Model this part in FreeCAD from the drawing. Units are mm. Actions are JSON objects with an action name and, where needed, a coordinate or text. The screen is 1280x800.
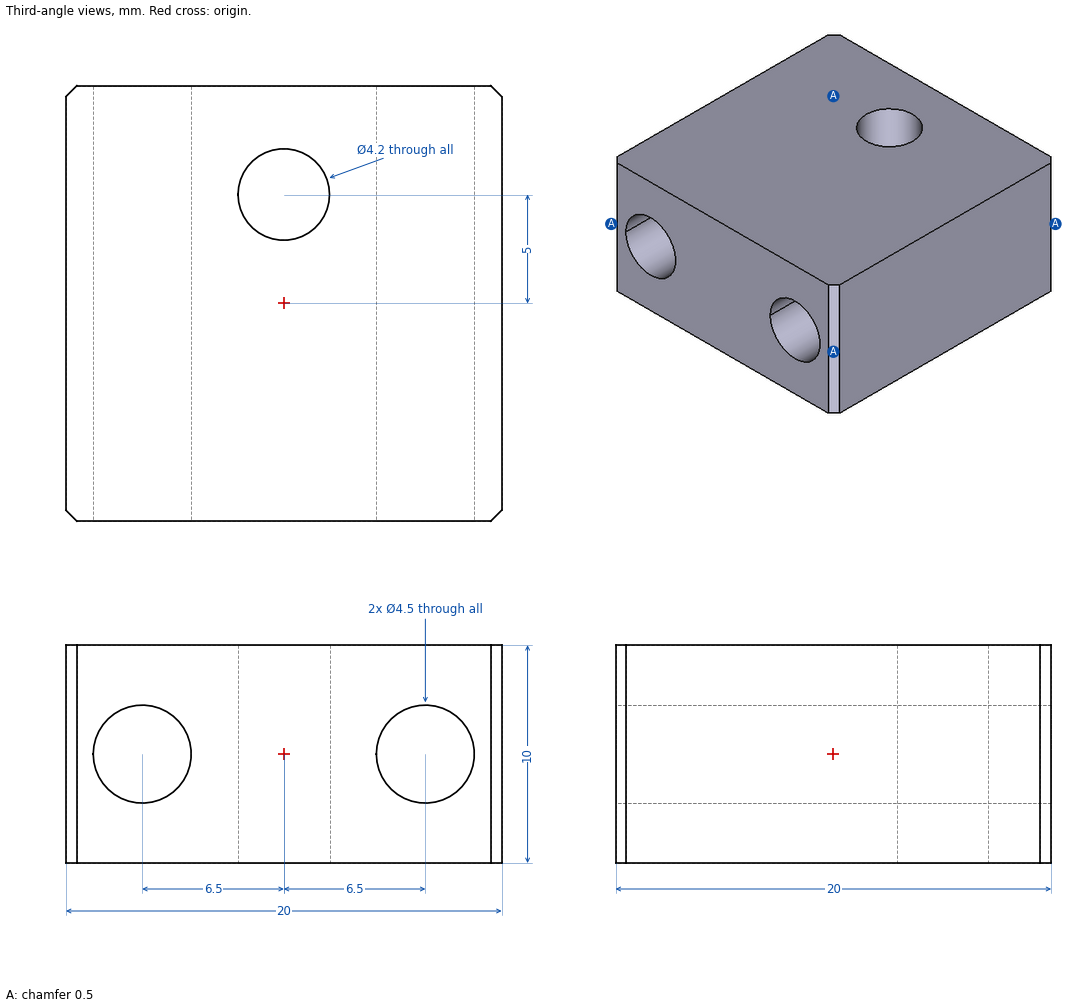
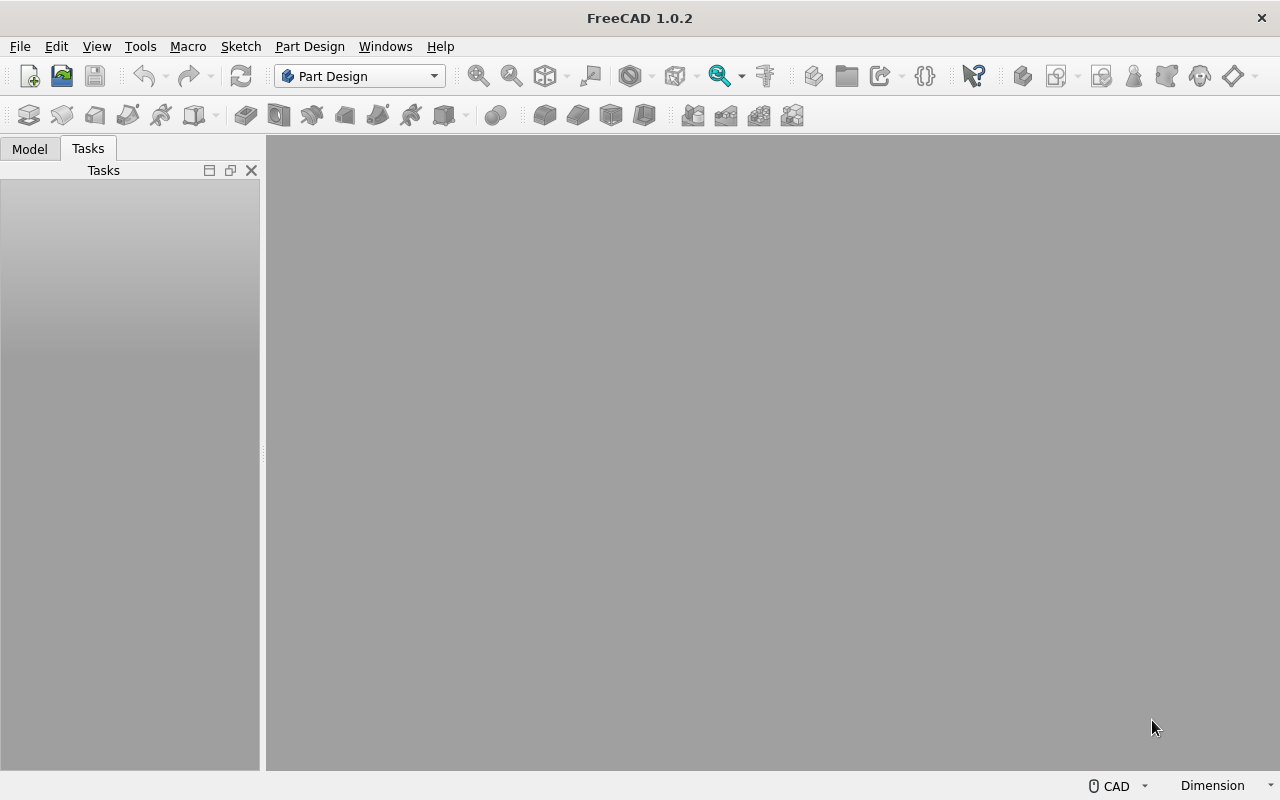
{"action": "key", "text": "ctrl+n"}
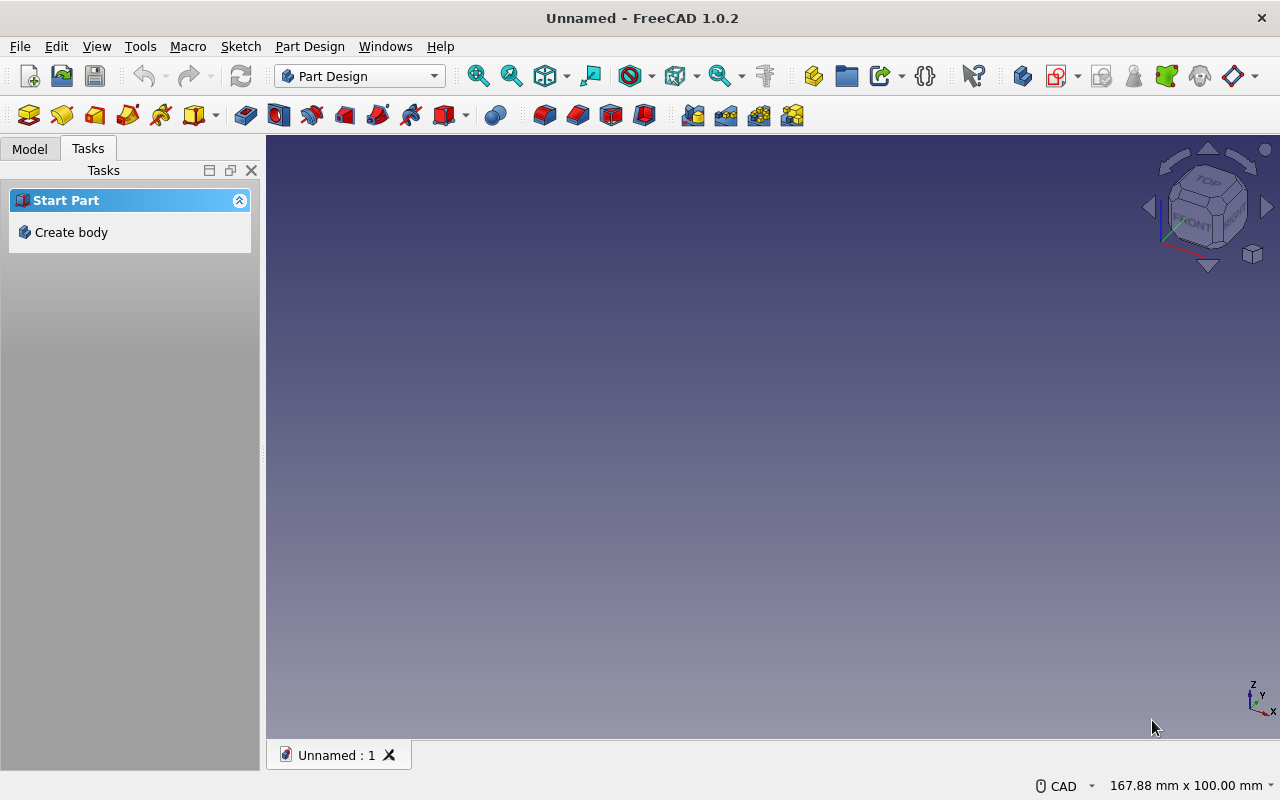
{"action": "left_click", "coordinate": [1056, 76]}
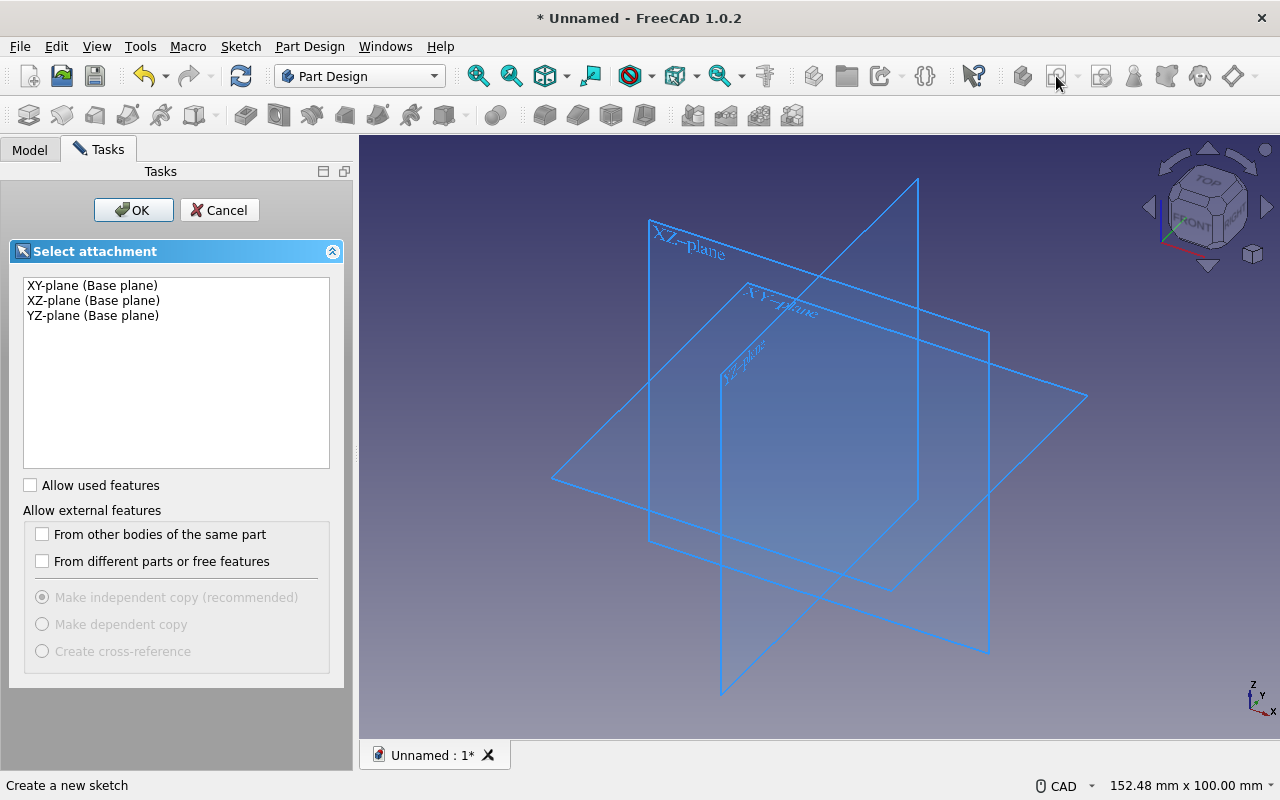
{"action": "left_click", "coordinate": [84, 300]}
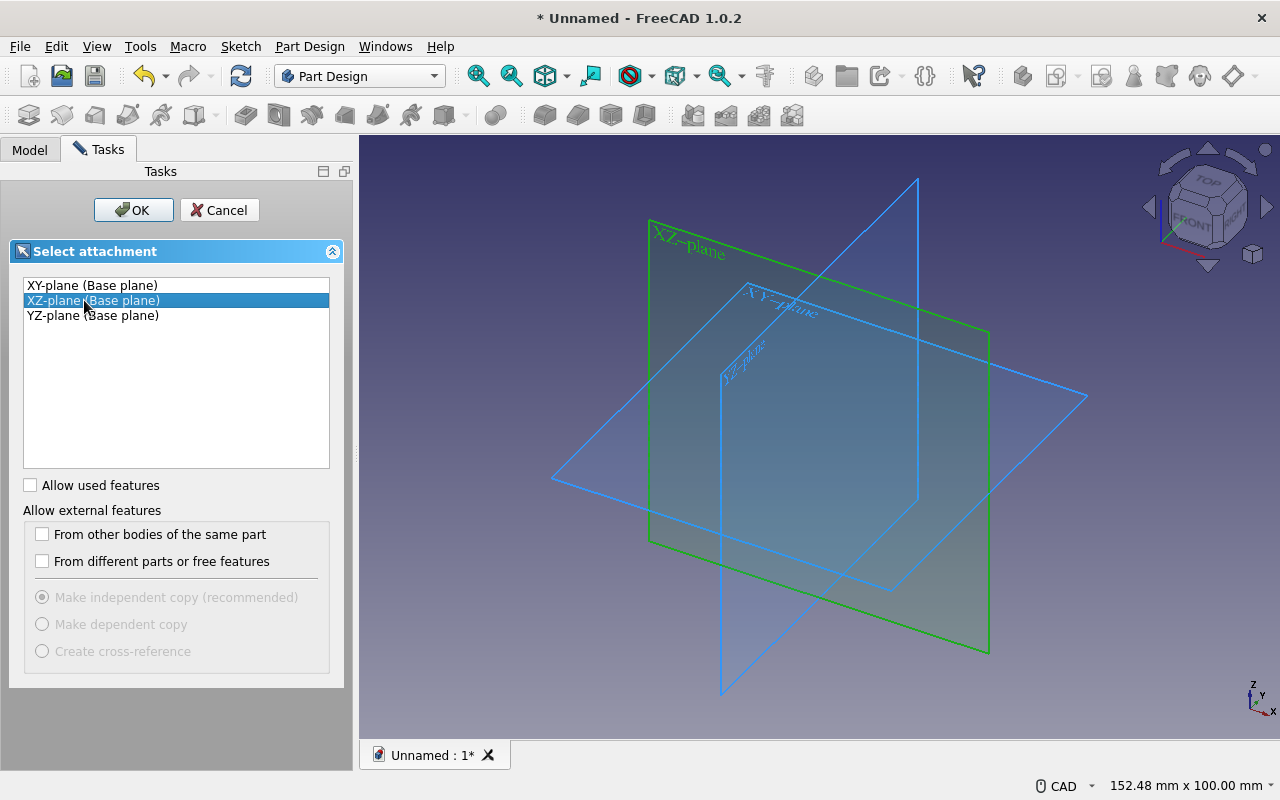
{"action": "left_click", "coordinate": [134, 210]}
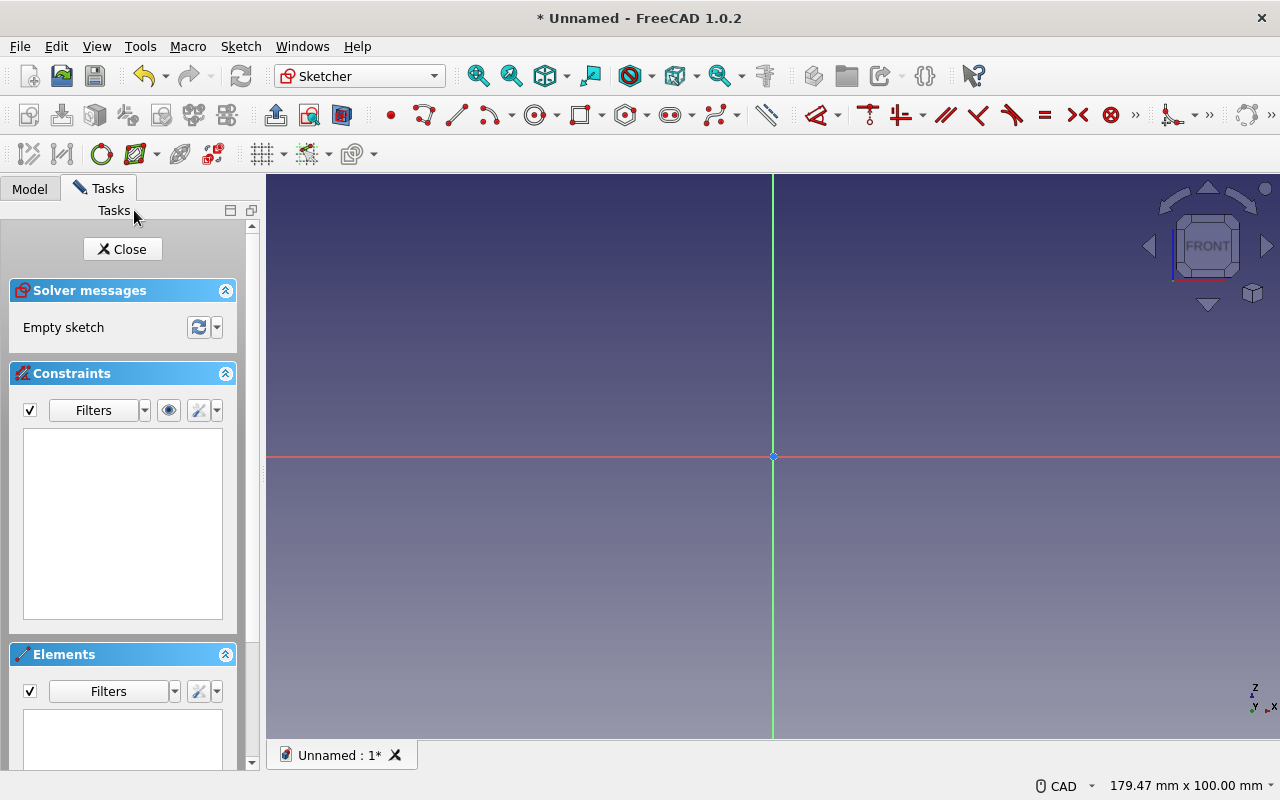
{"action": "scroll", "coordinate": [790, 456], "scroll_direction": "up", "scroll_amount": 8}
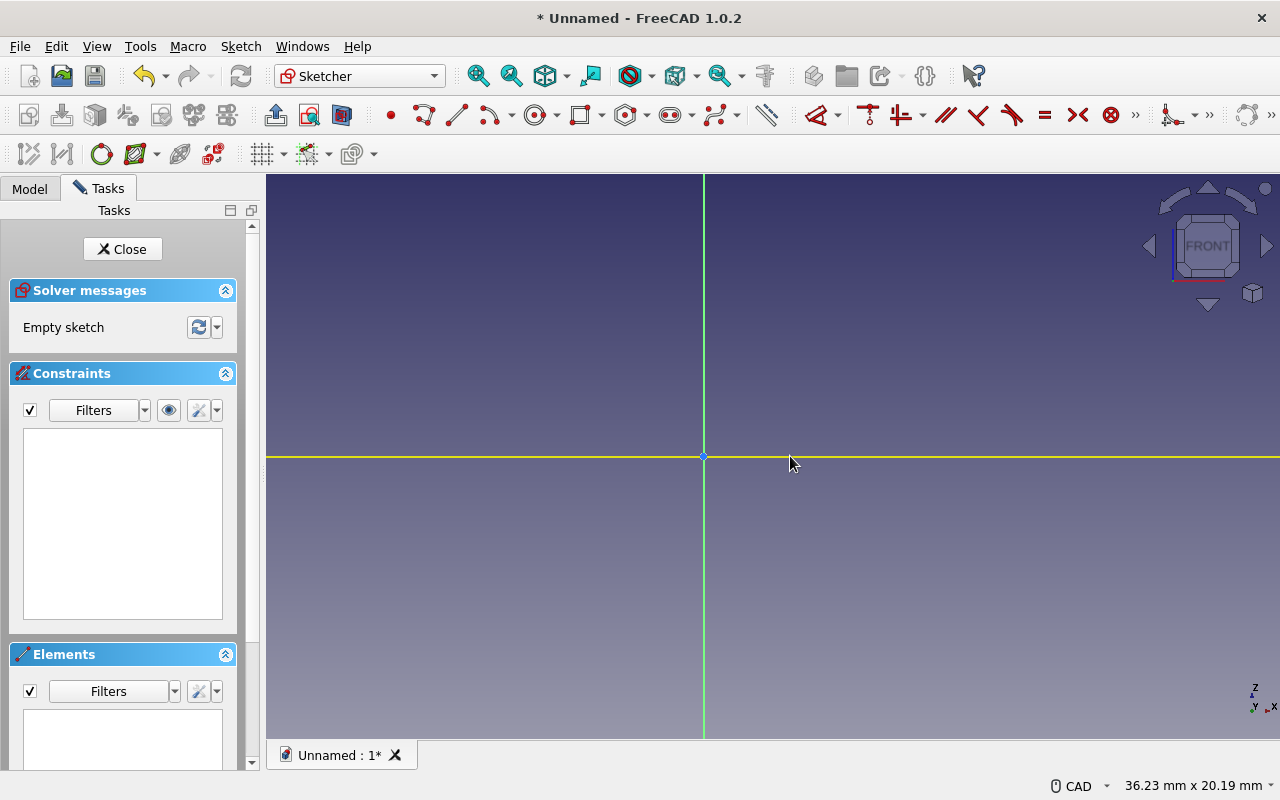
{"action": "key", "text": "g v"}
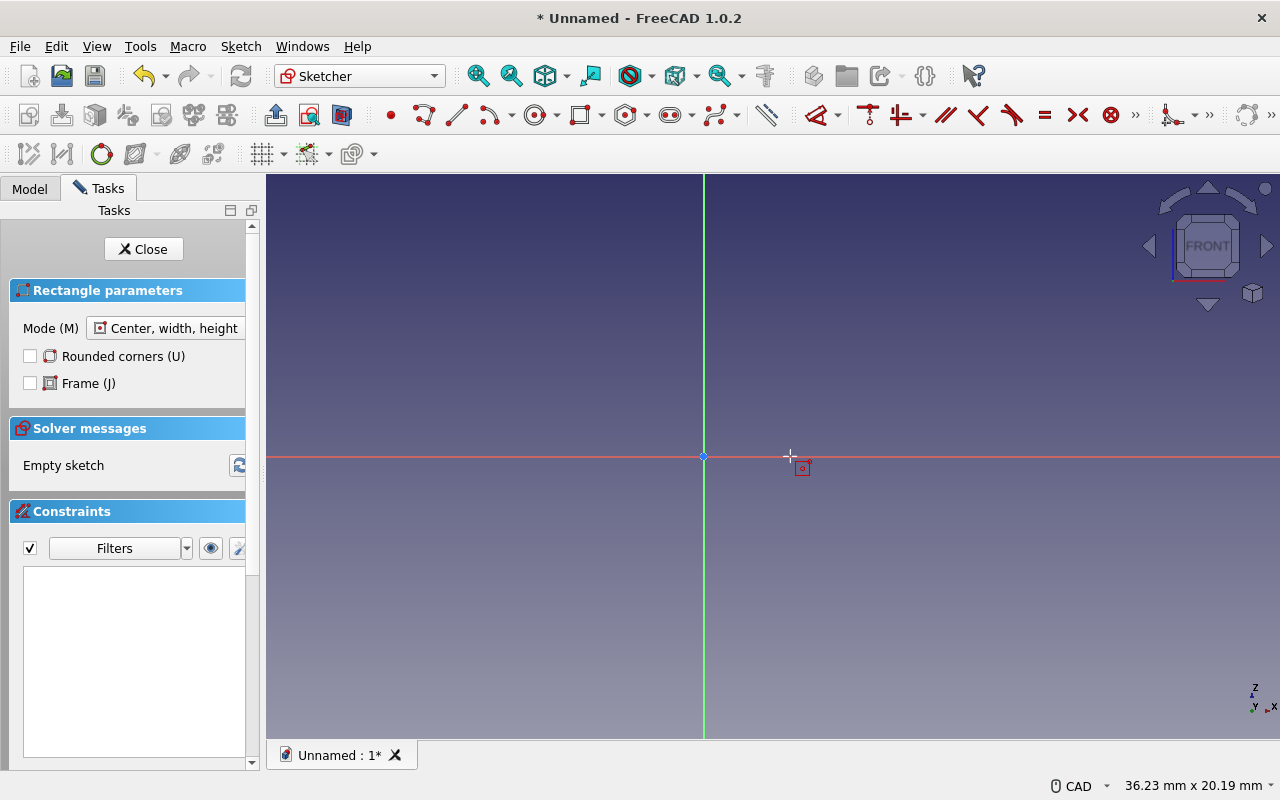
{"action": "left_click", "coordinate": [704, 456]}
{"action": "left_click", "coordinate": [984, 317]}
{"action": "key", "text": "Escape"}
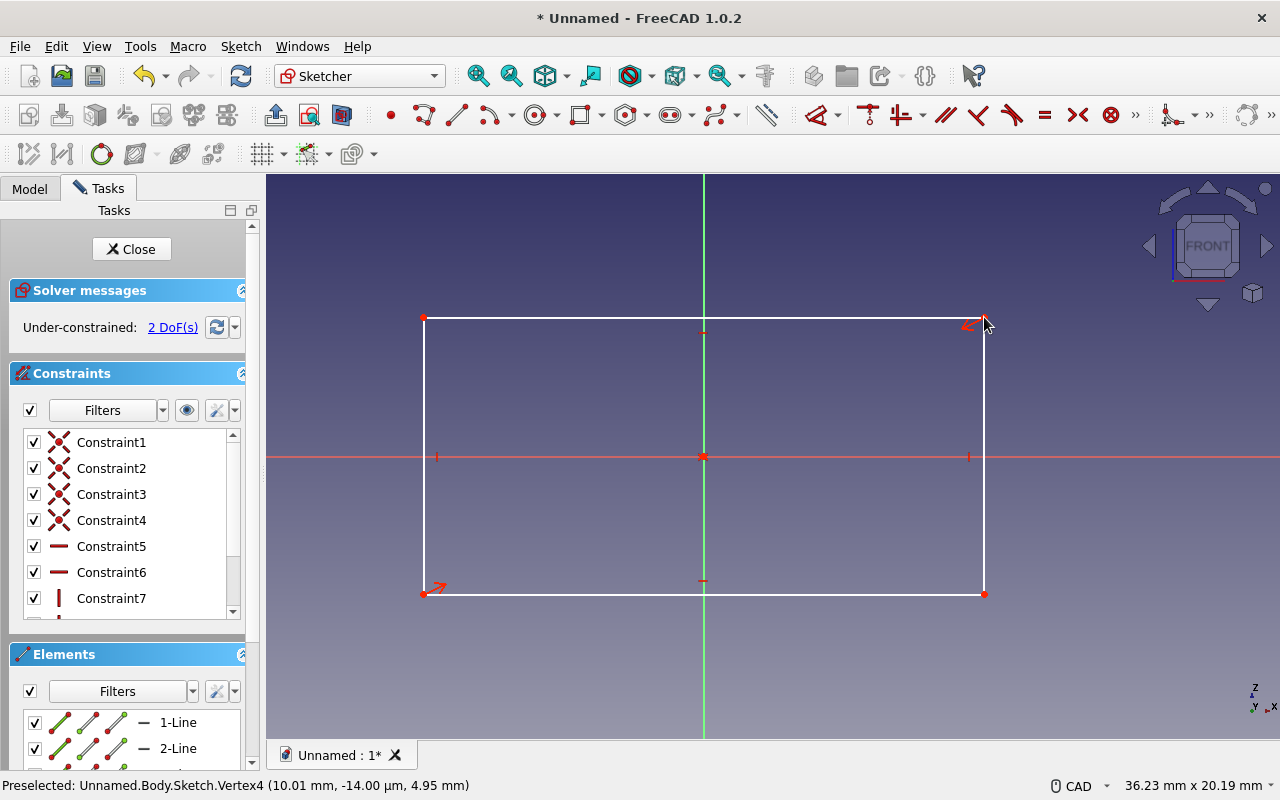
{"action": "key", "text": "d"}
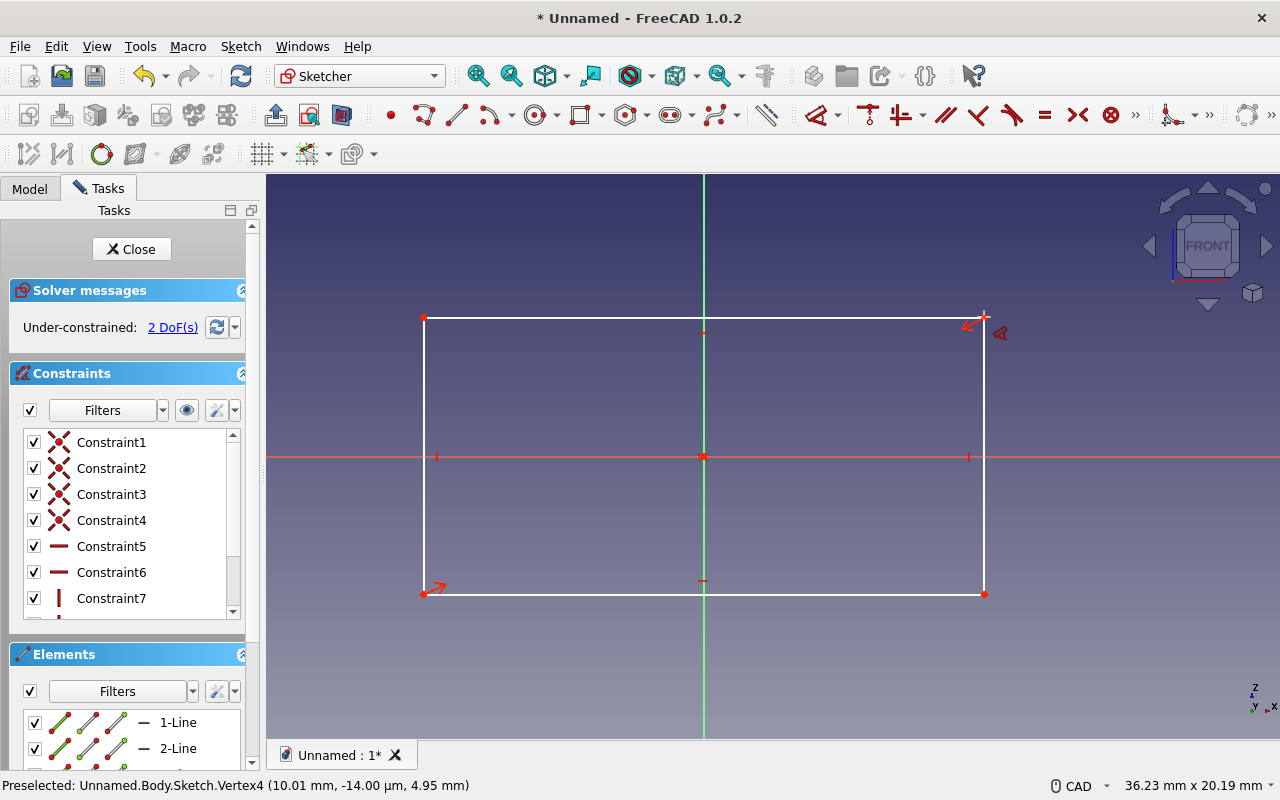
{"action": "left_click", "coordinate": [592, 595]}
{"action": "left_click", "coordinate": [575, 629]}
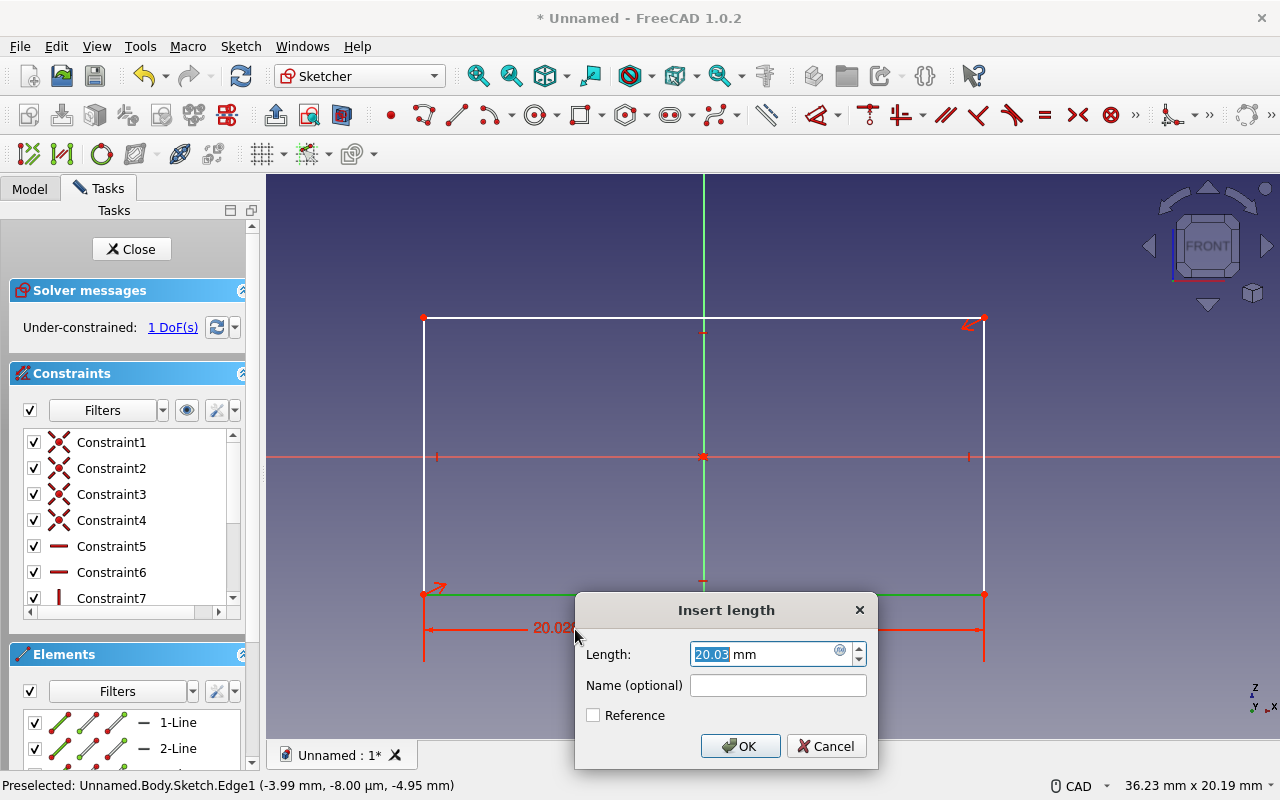
{"action": "type", "text": "20"}
{"action": "key", "text": "Return"}